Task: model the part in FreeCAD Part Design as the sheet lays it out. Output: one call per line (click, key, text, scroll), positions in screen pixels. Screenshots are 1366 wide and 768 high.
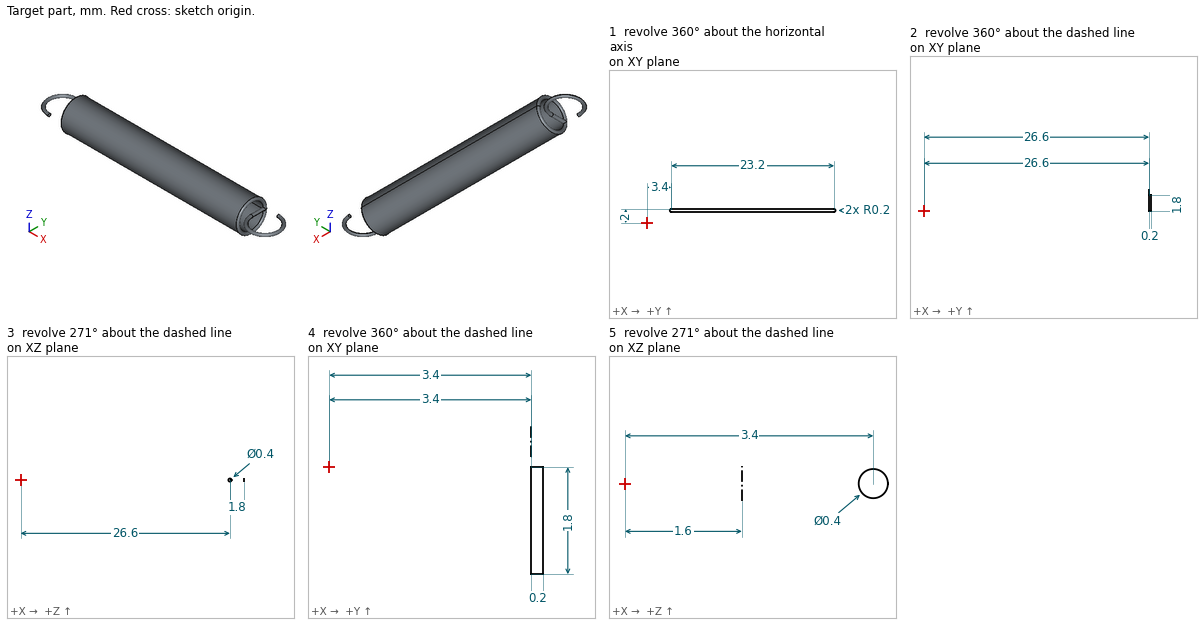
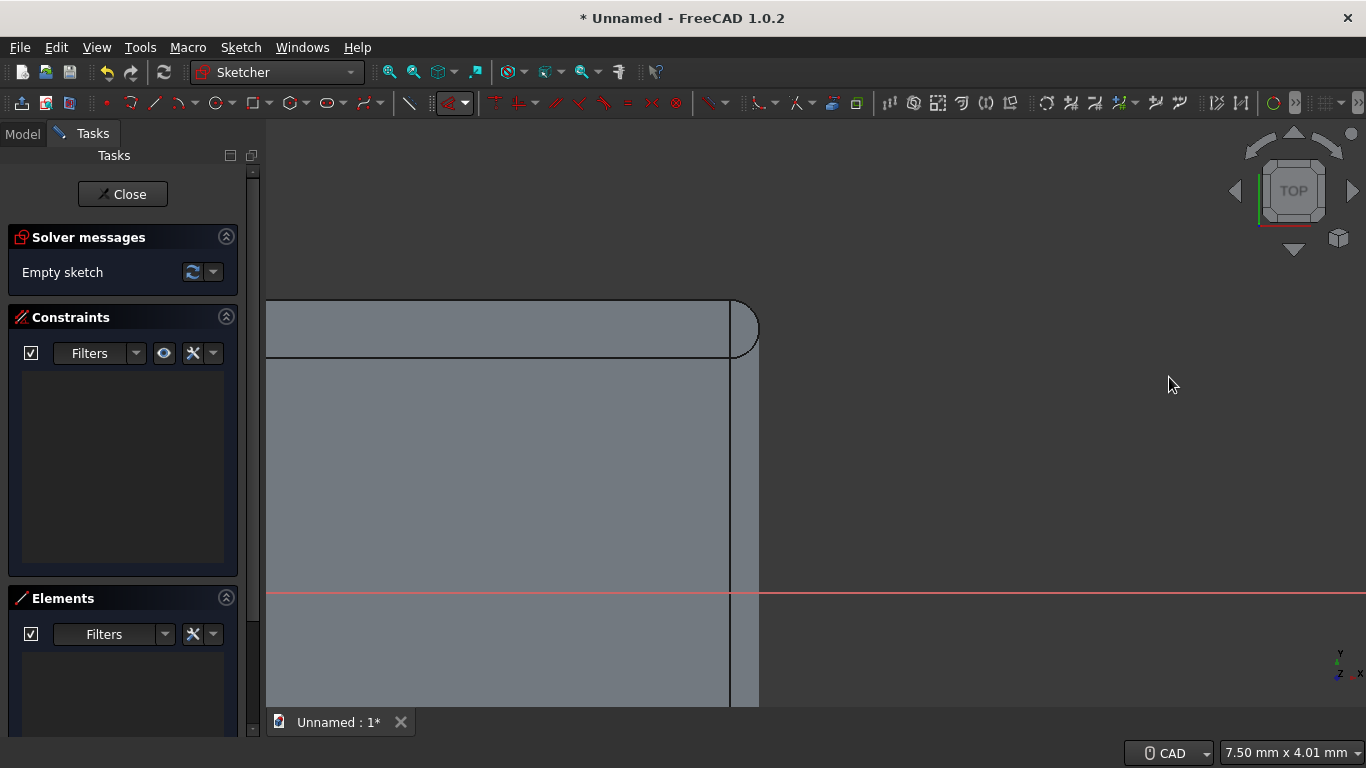
click(254, 104)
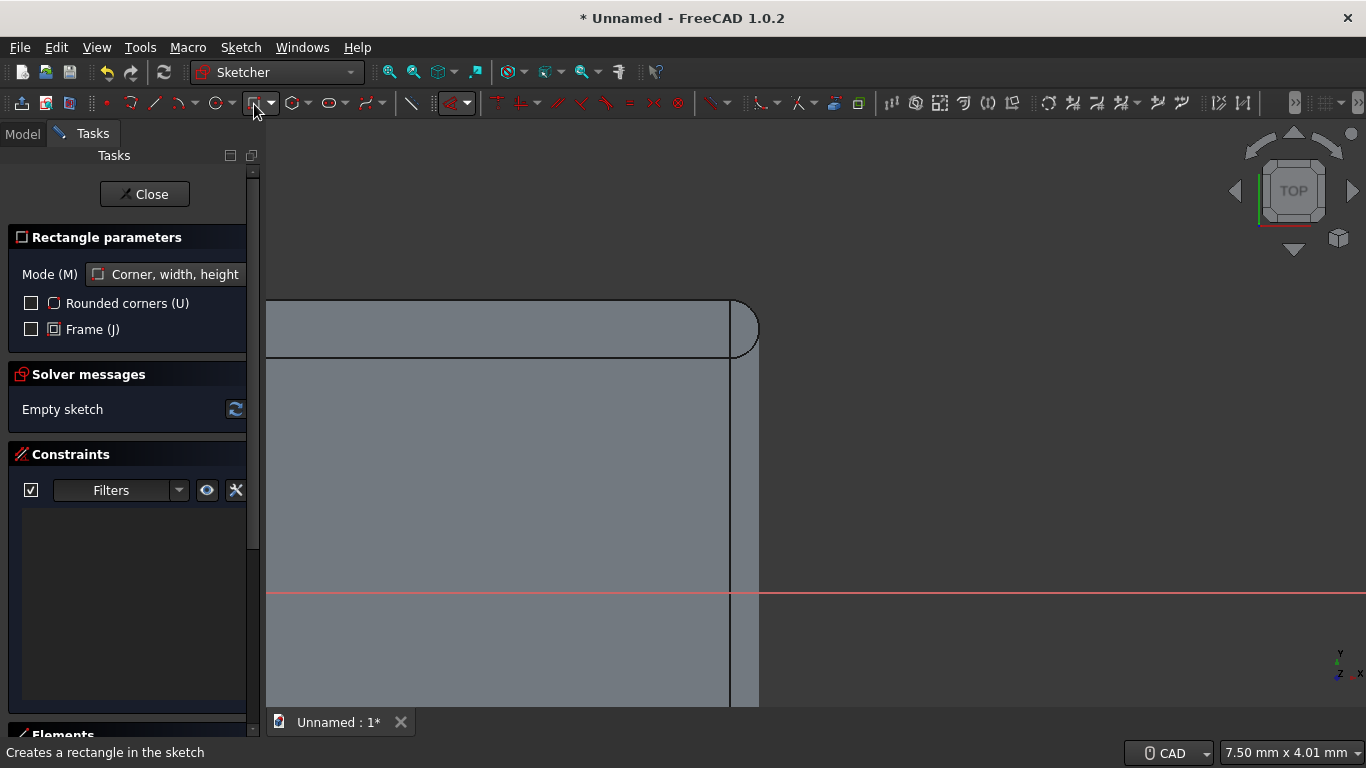
click(730, 329)
click(759, 593)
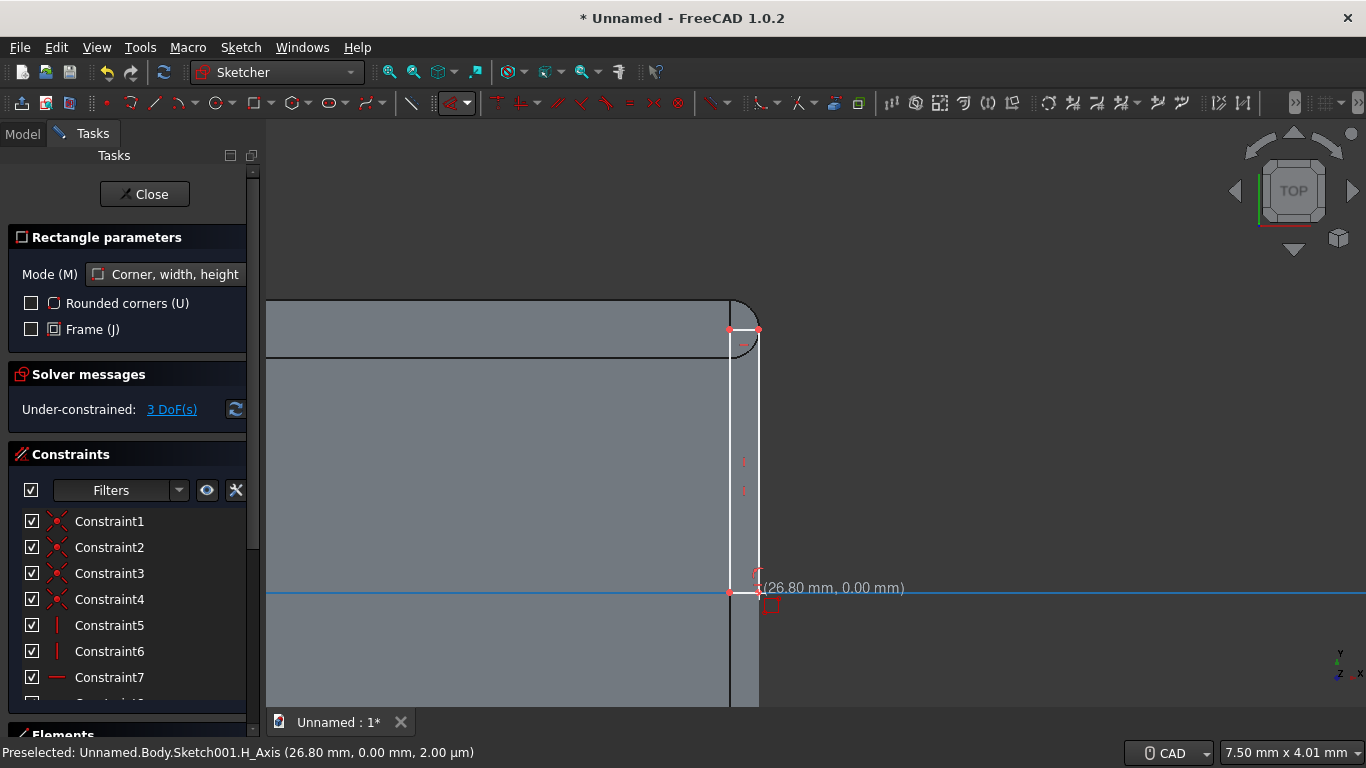
click(156, 104)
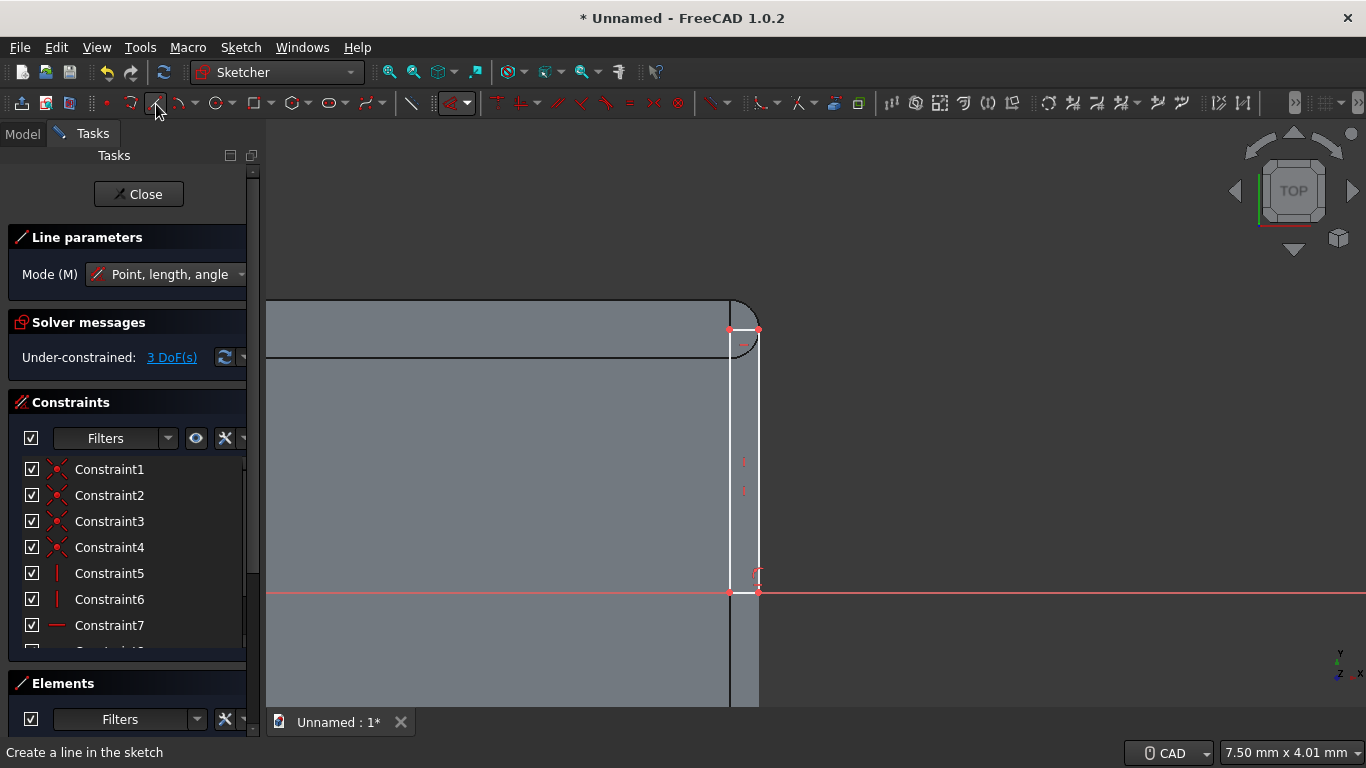
click(730, 303)
click(730, 224)
key(Escape)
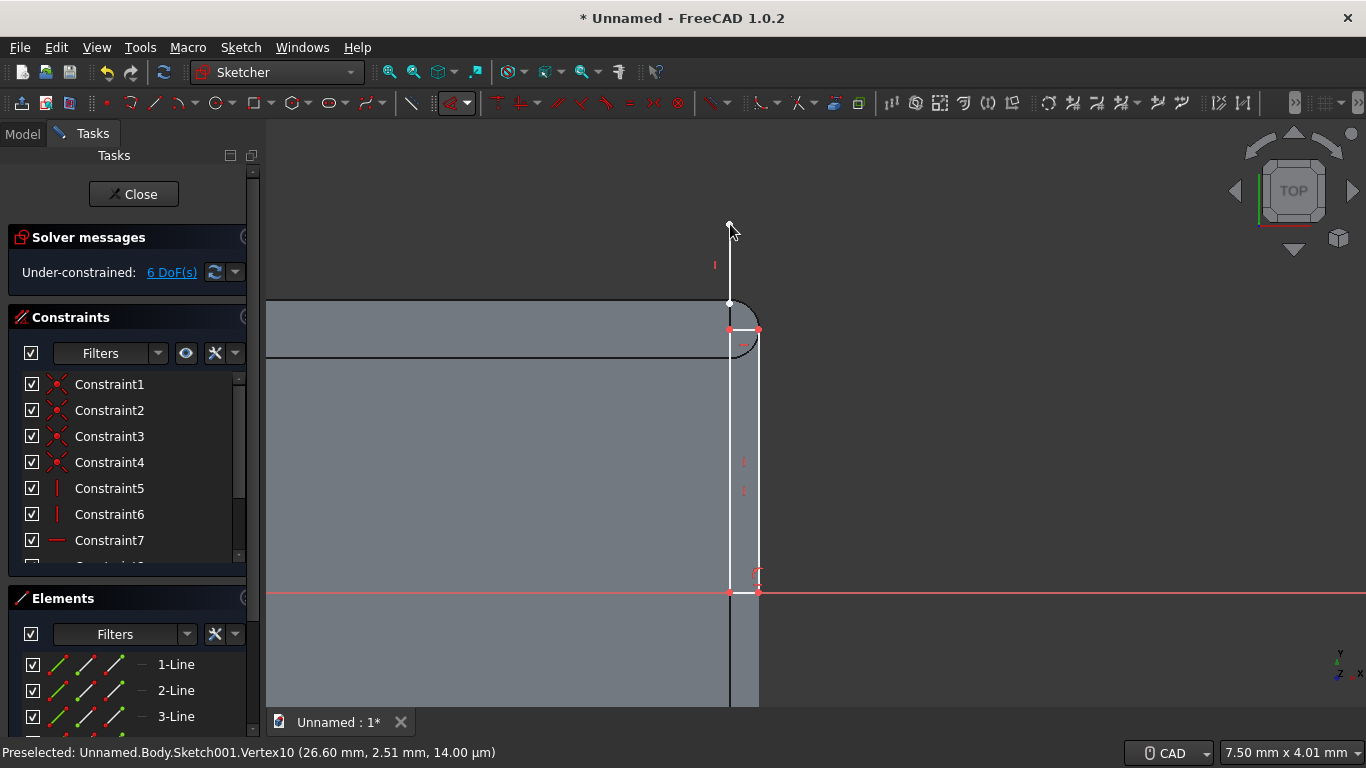
click(730, 280)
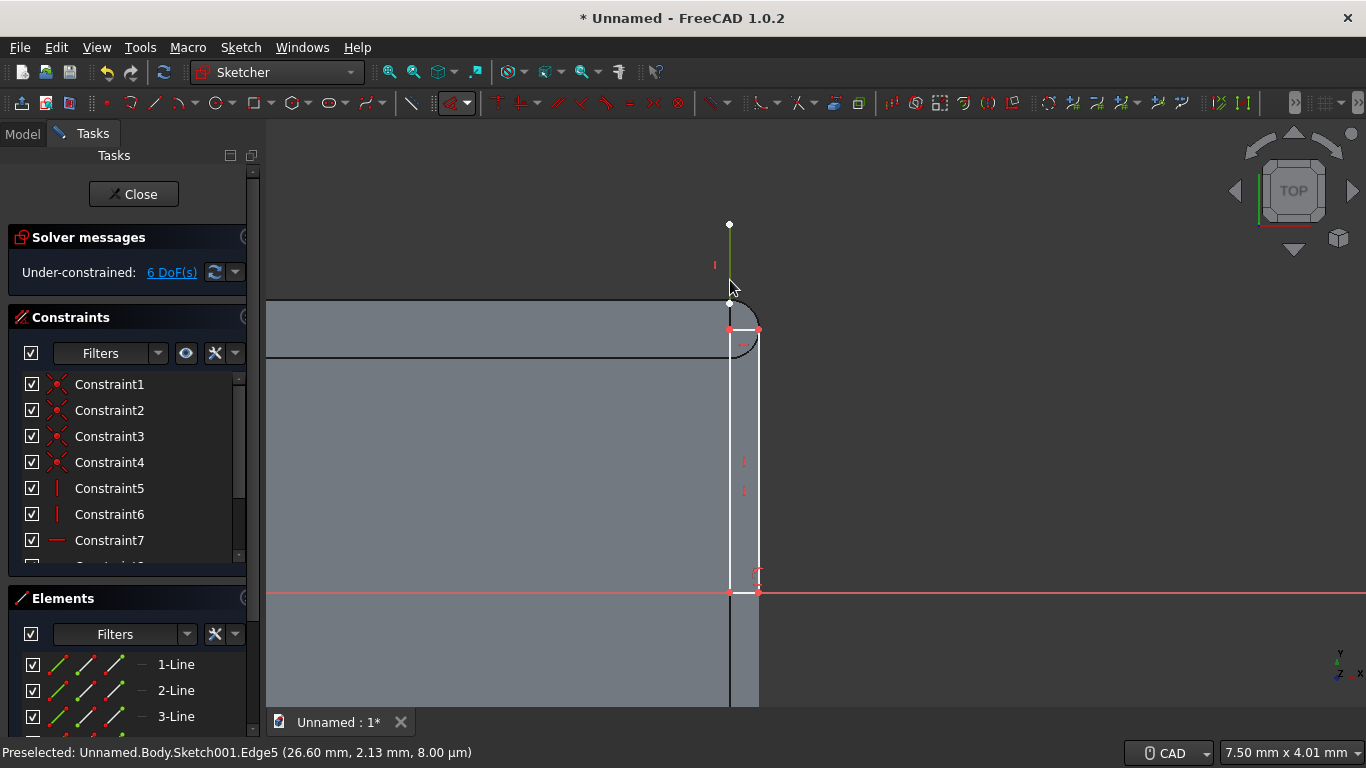
click(412, 104)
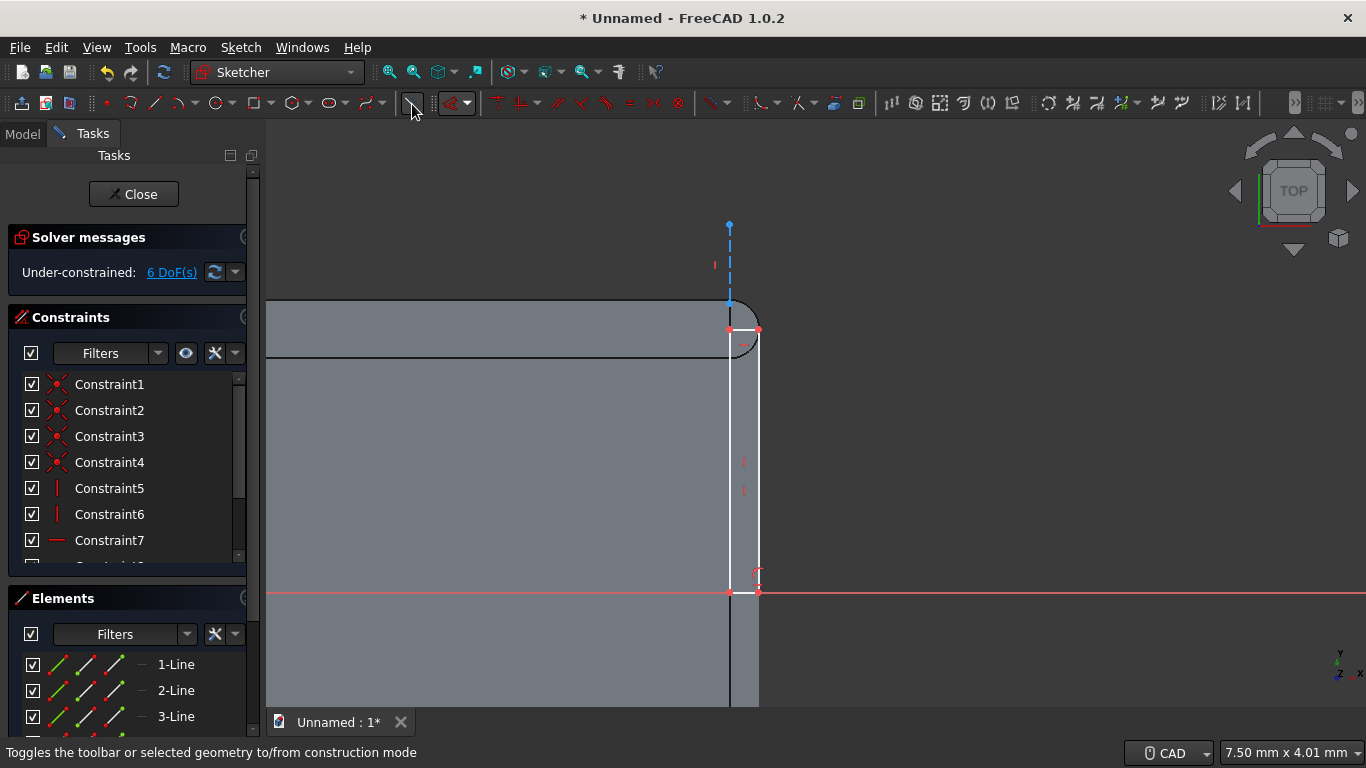
click(730, 409)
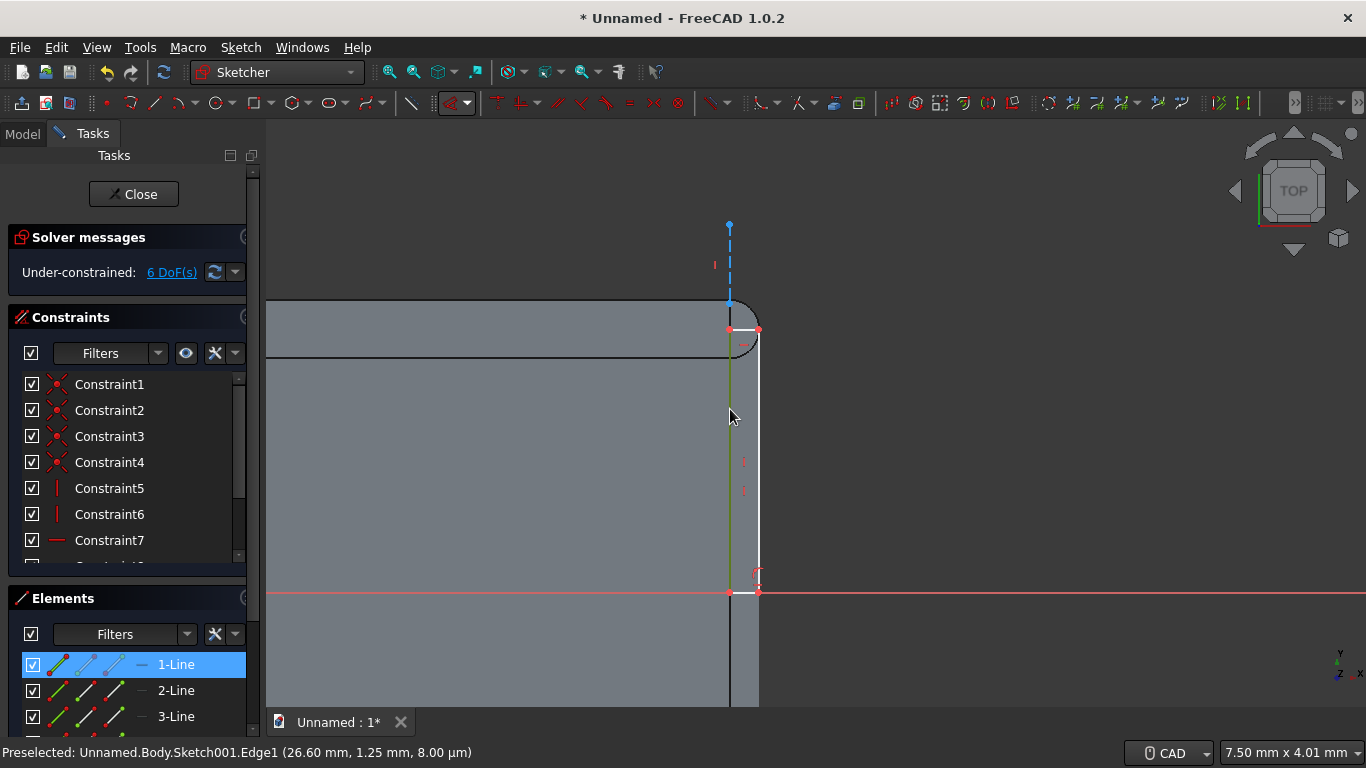
key(i)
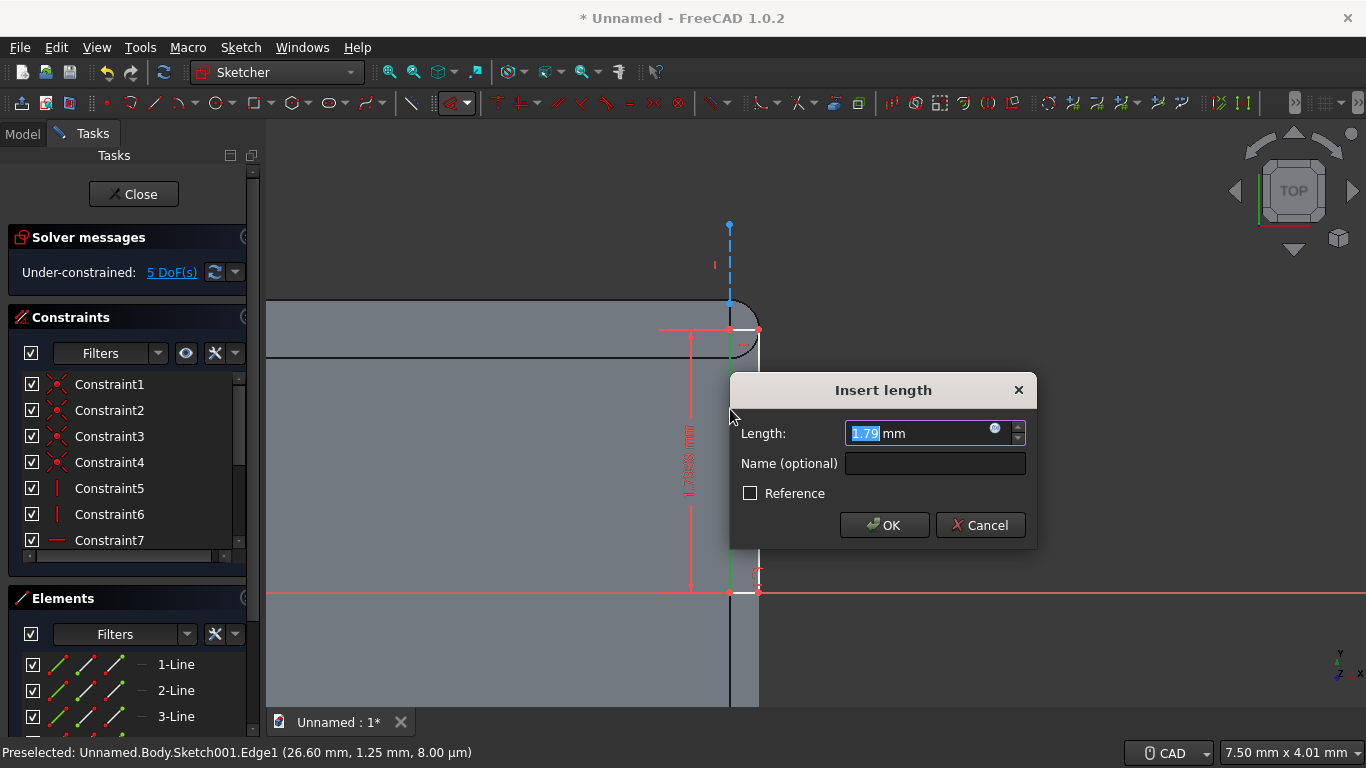
text(1.8)
key(Return)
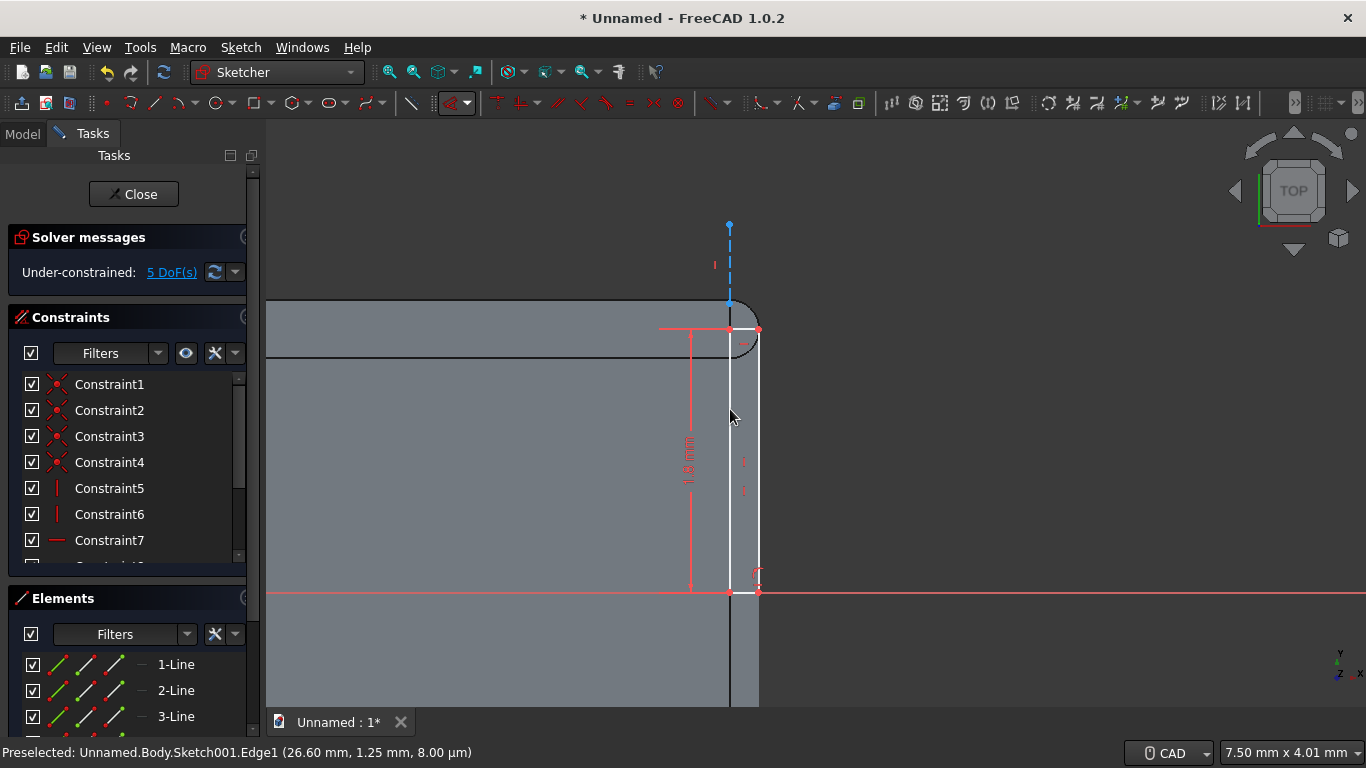
scroll(742, 593, up, 2)